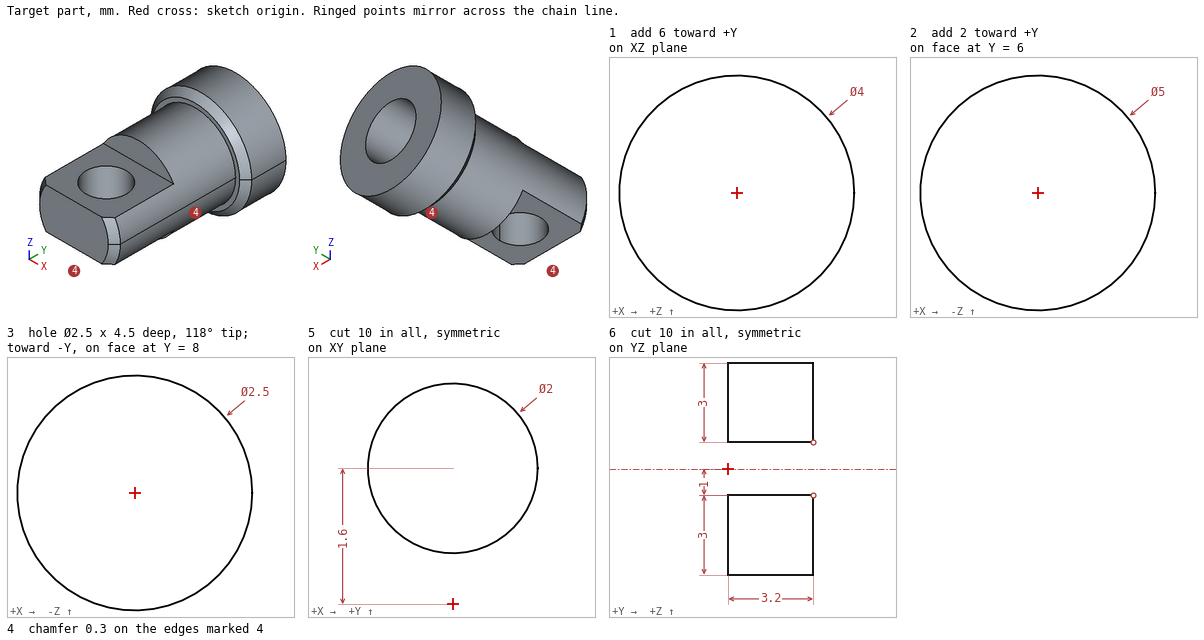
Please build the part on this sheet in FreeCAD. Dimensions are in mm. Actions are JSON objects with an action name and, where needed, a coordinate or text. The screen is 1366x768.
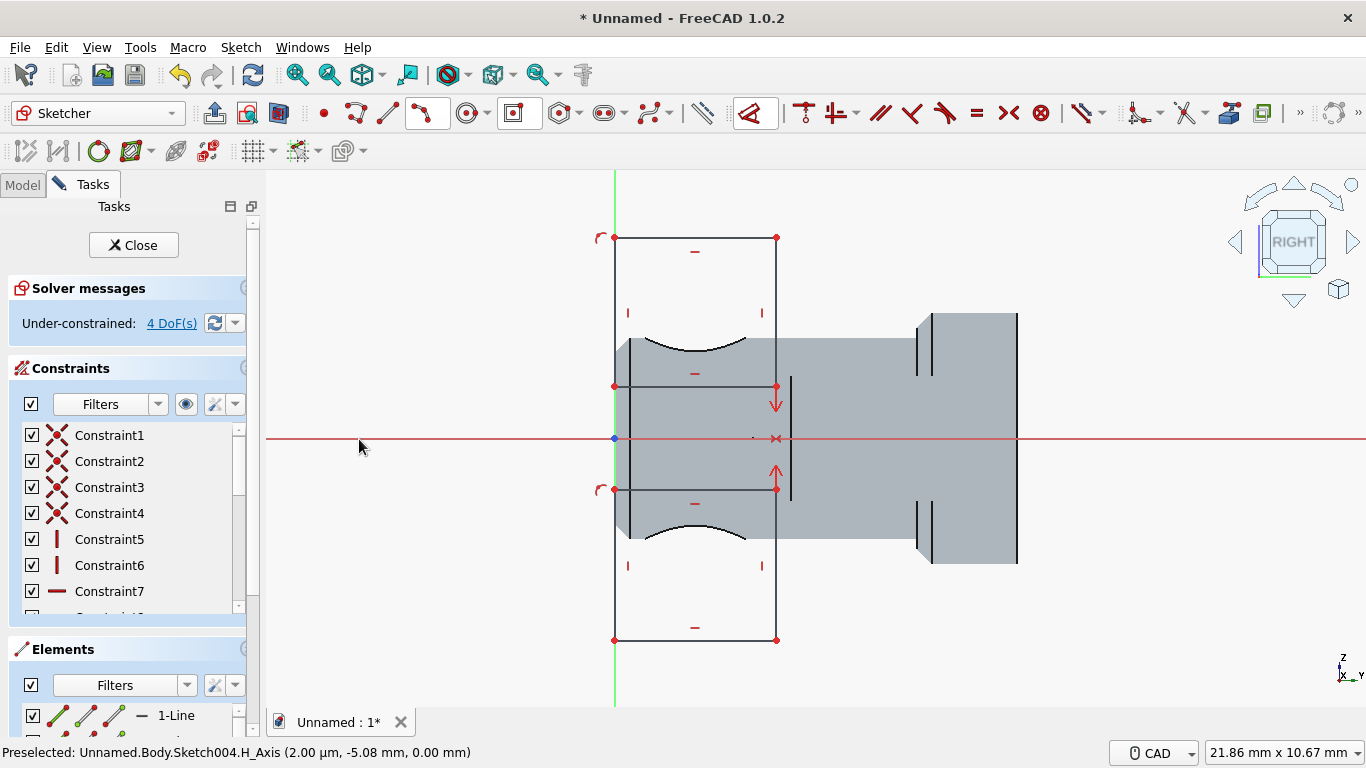
{"action": "left_click", "coordinate": [615, 535]}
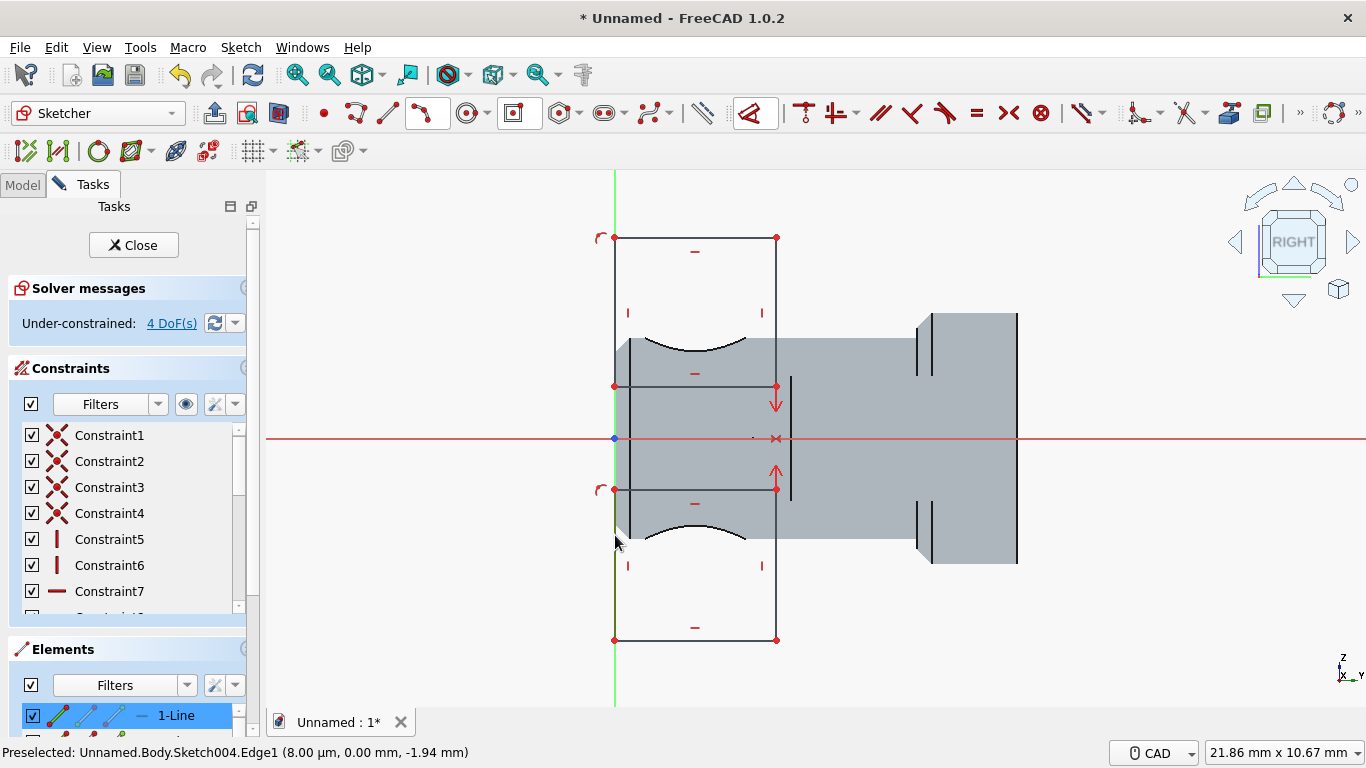
{"action": "key", "text": "i"}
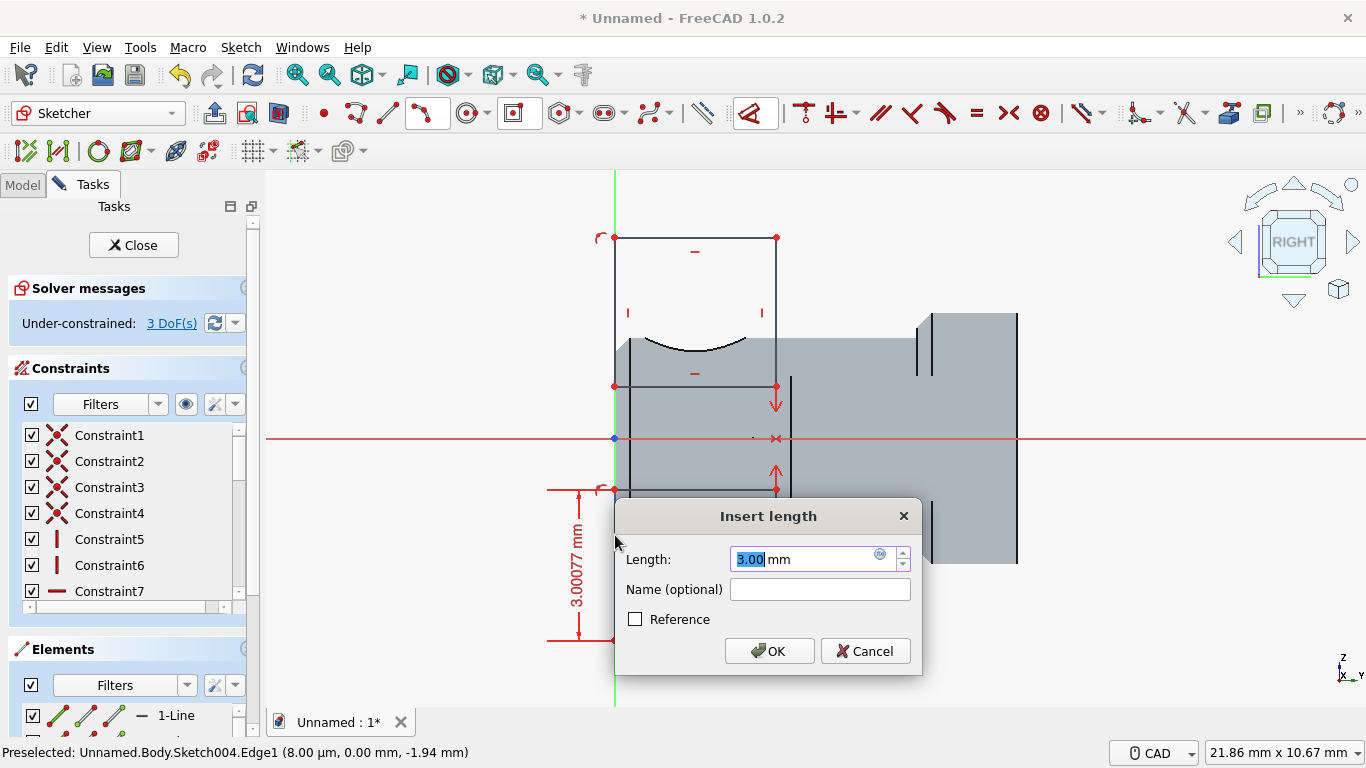
{"action": "type", "text": "3"}
{"action": "key", "text": "Return"}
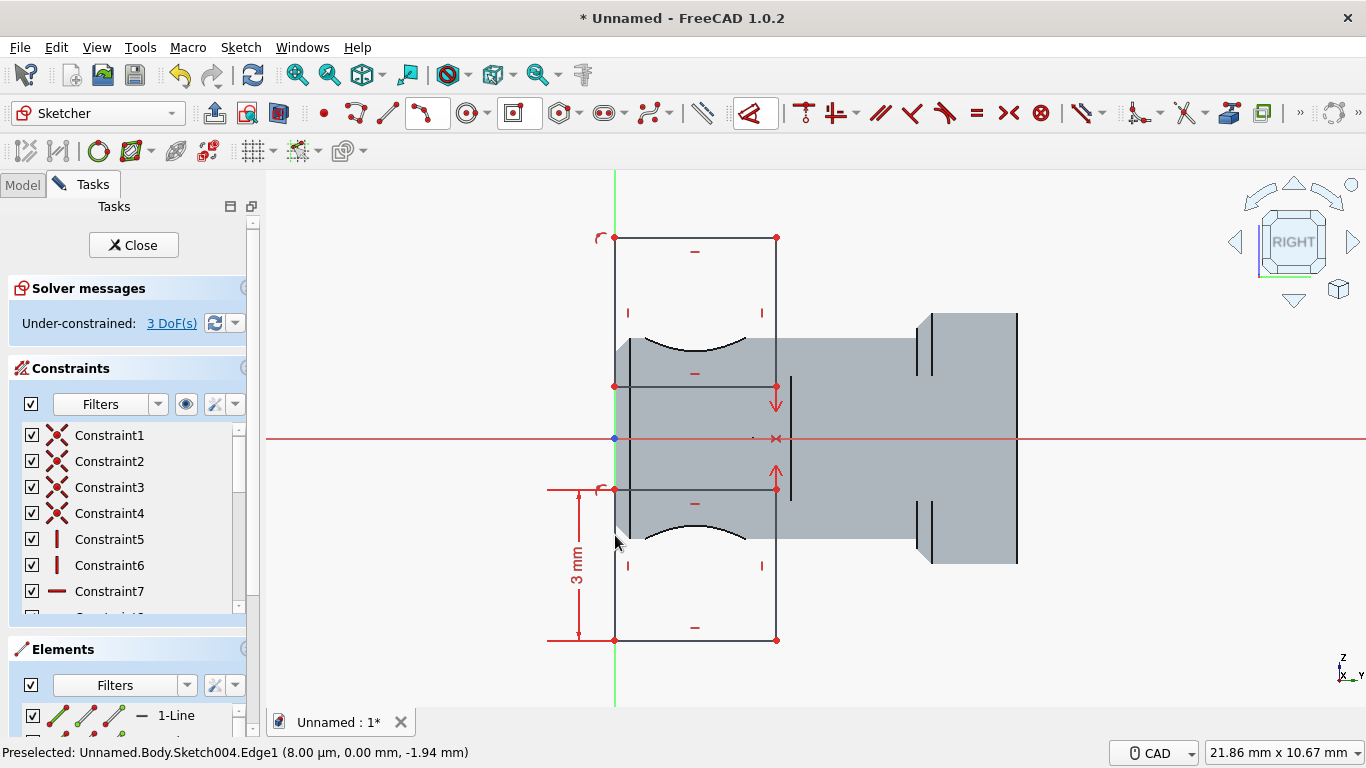
{"action": "left_click", "coordinate": [615, 283]}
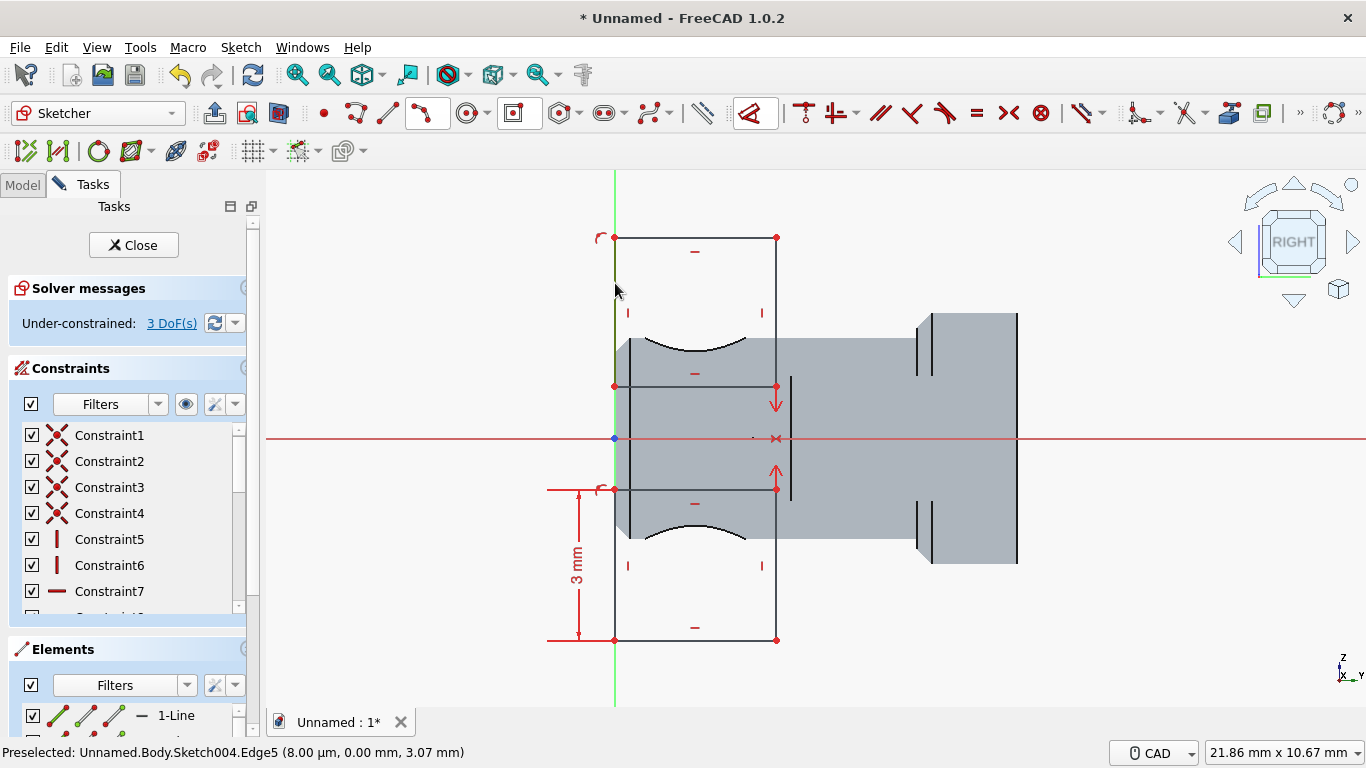
{"action": "left_click", "coordinate": [772, 114]}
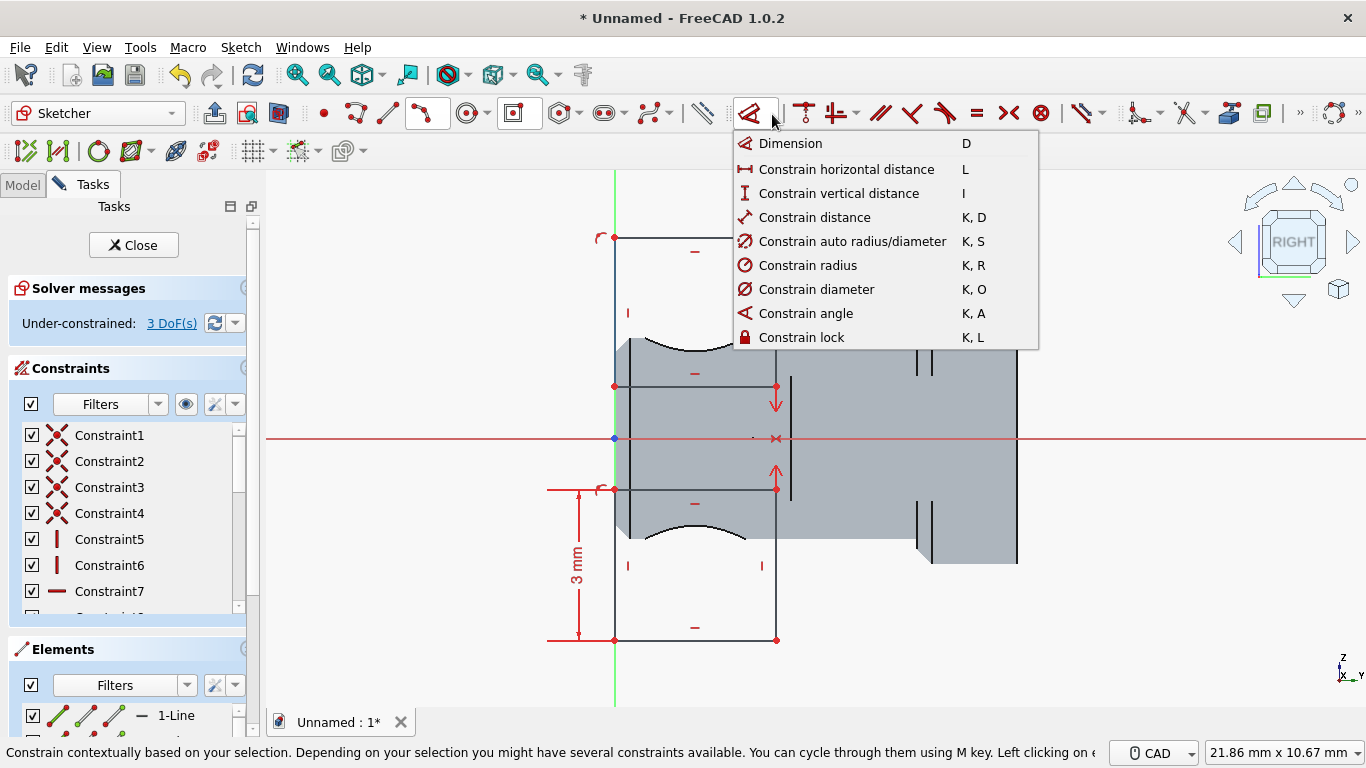
{"action": "left_click", "coordinate": [886, 193]}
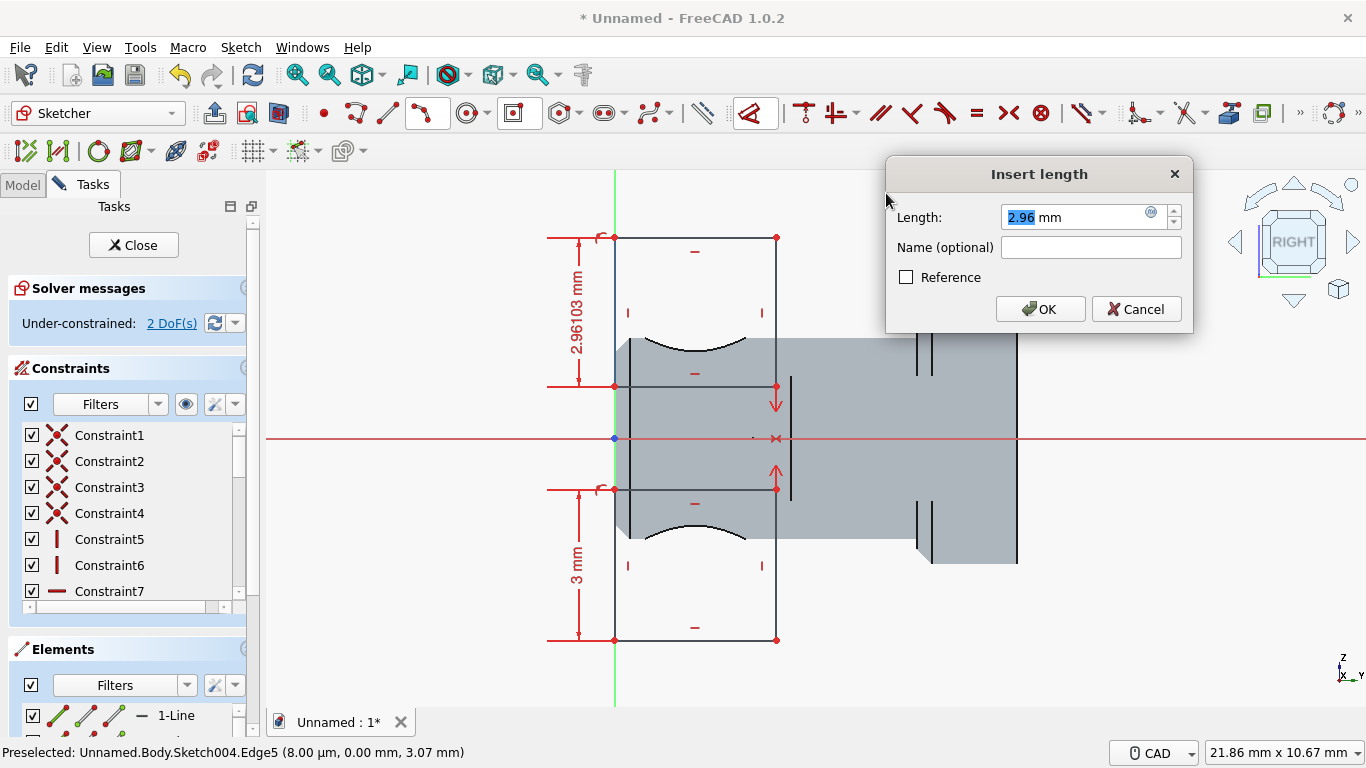
{"action": "type", "text": "3"}
{"action": "key", "text": "Return"}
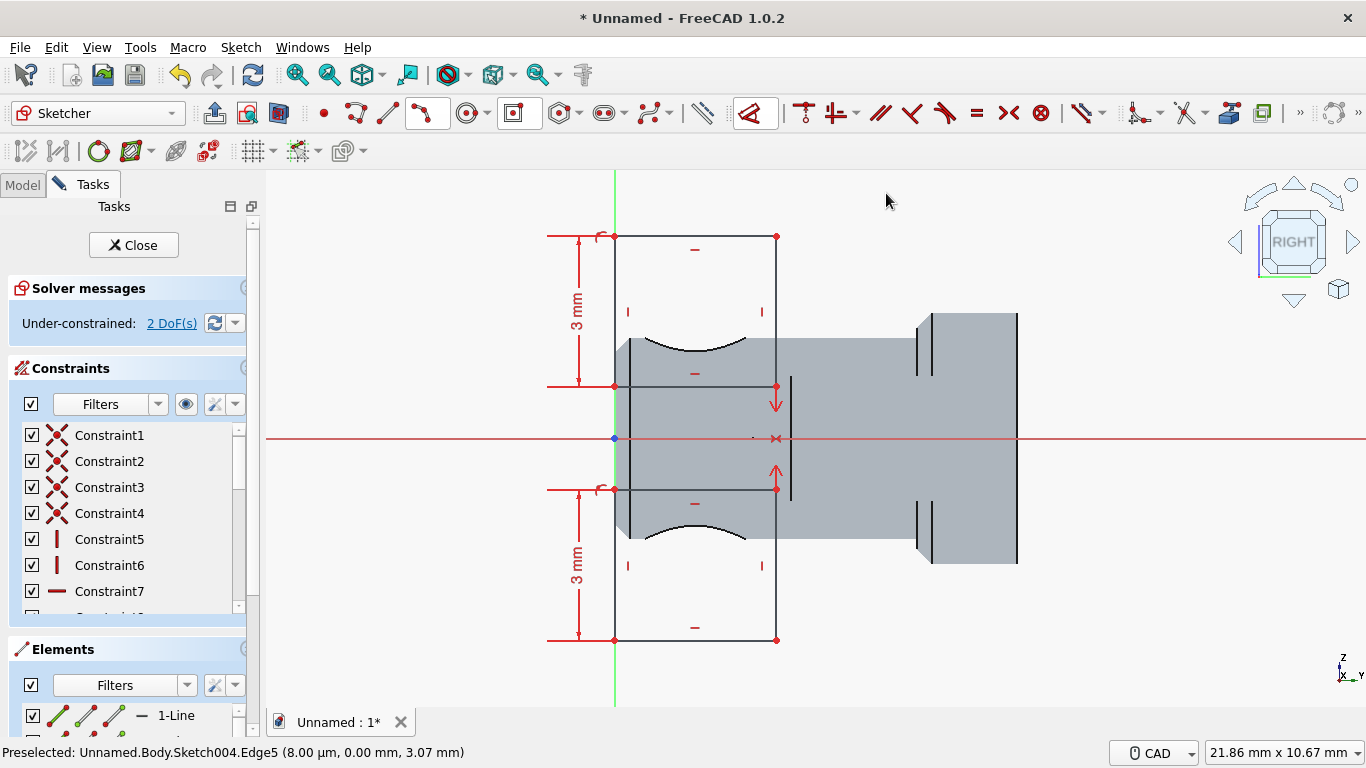
{"action": "left_click", "coordinate": [615, 490]}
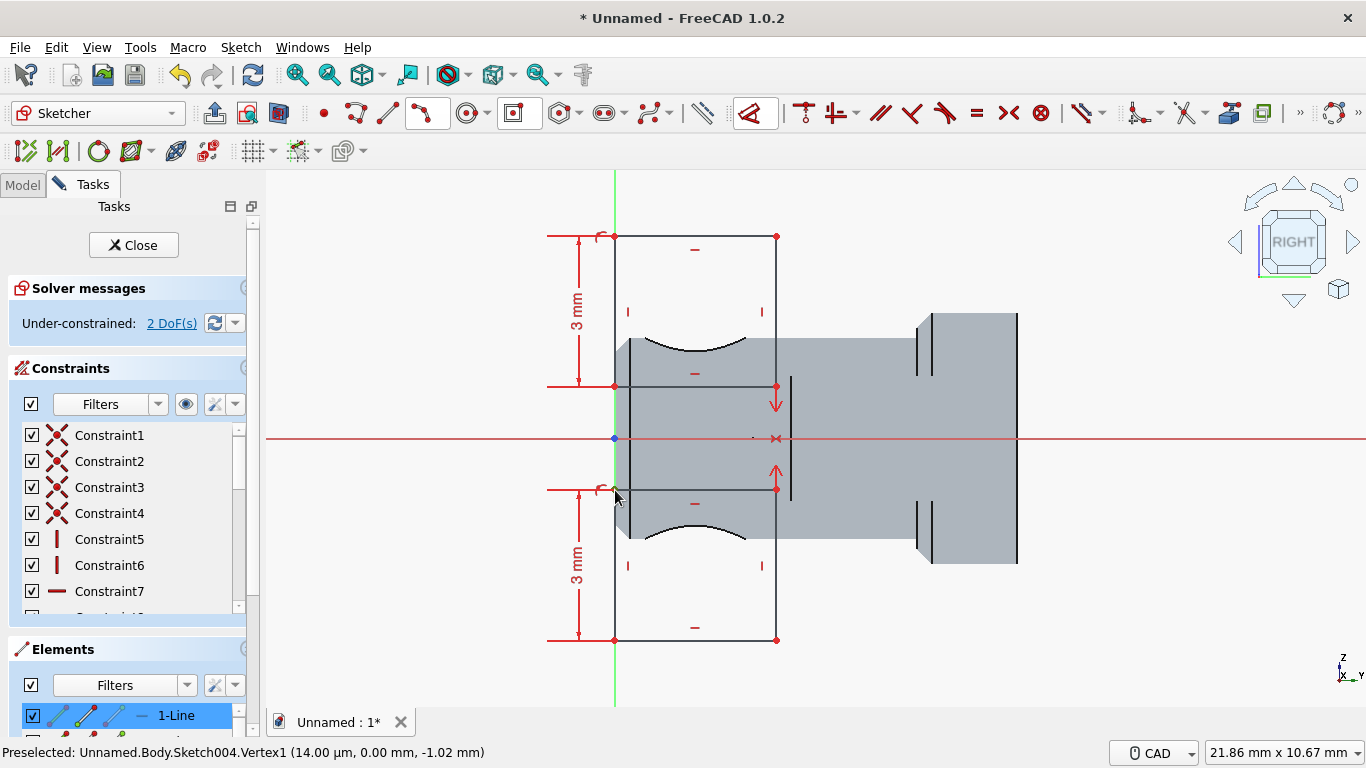
{"action": "key", "text": "i"}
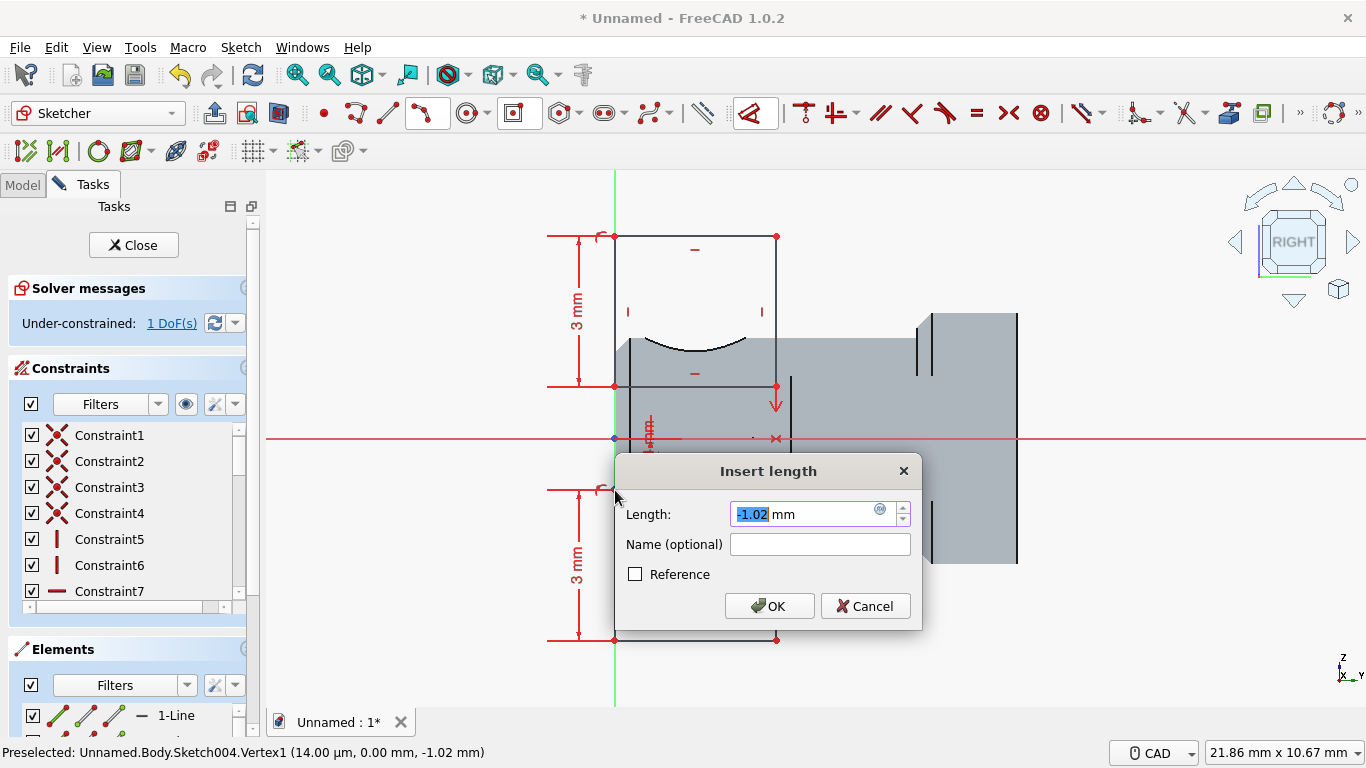
{"action": "type", "text": "-1"}
{"action": "key", "text": "Return"}